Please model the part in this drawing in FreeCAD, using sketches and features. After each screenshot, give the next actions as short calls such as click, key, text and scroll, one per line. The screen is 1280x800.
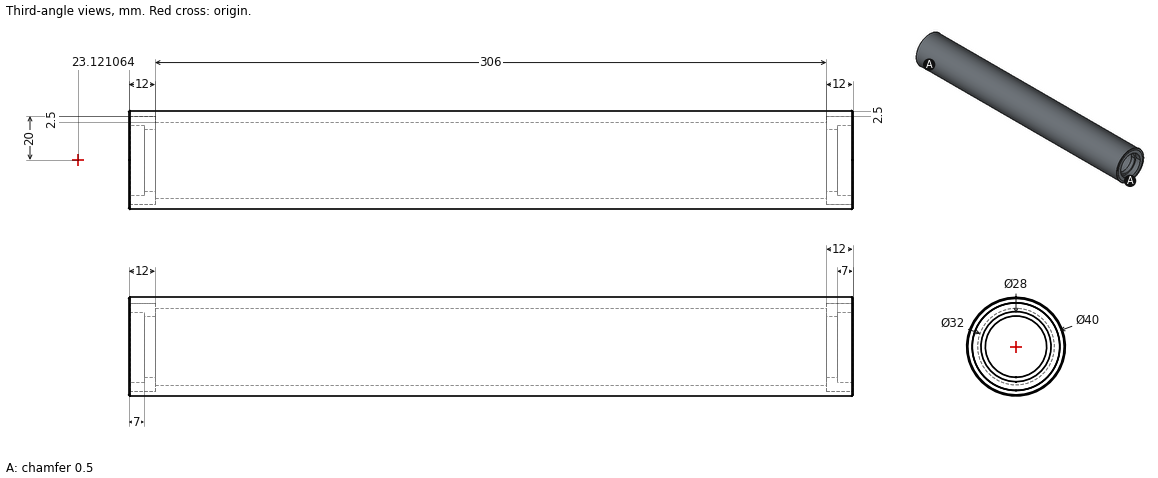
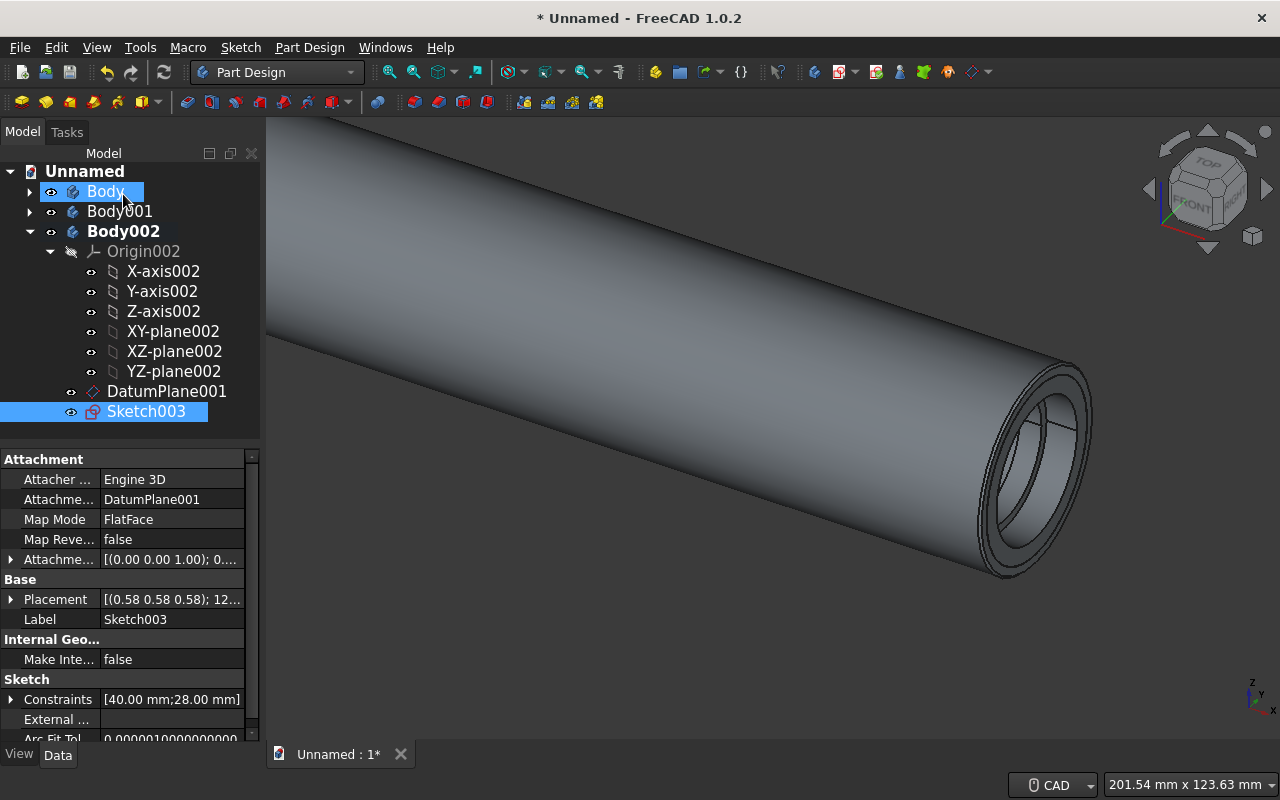
click(22, 102)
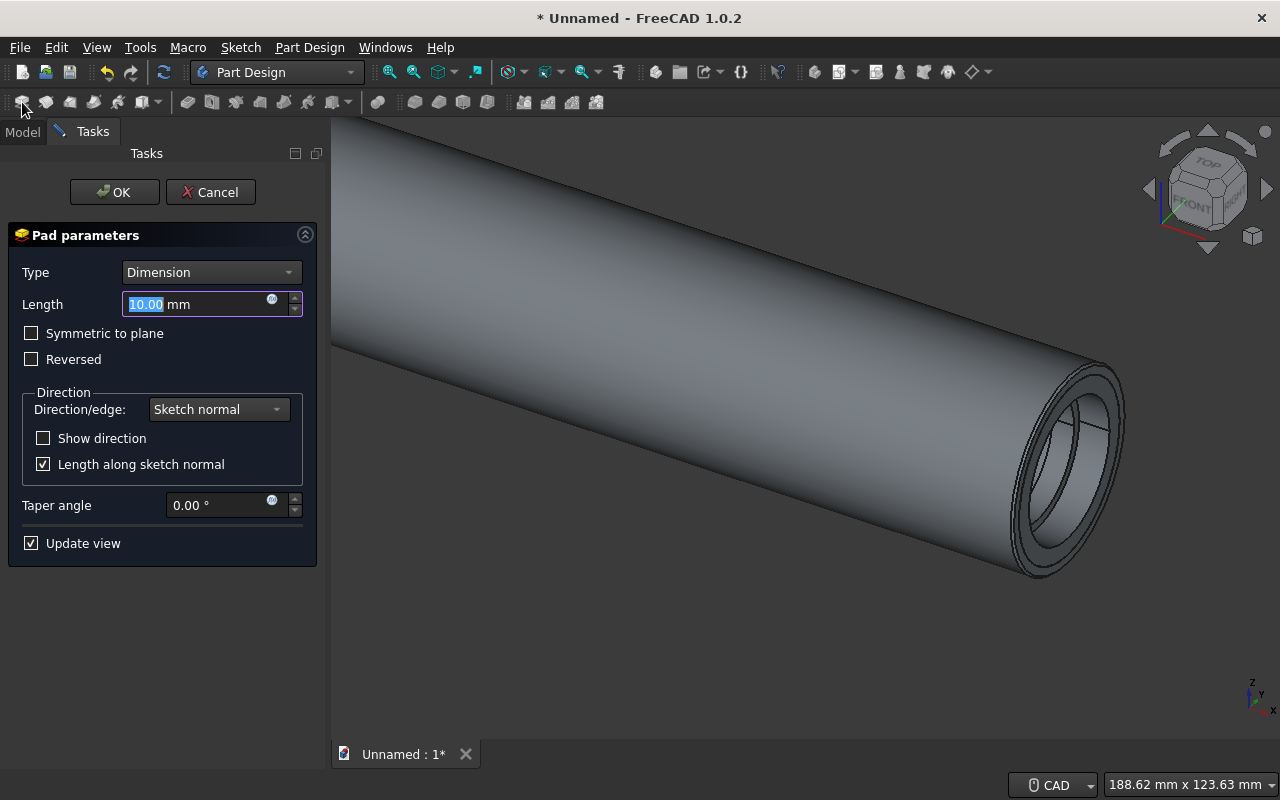
text(12)
key(Tab)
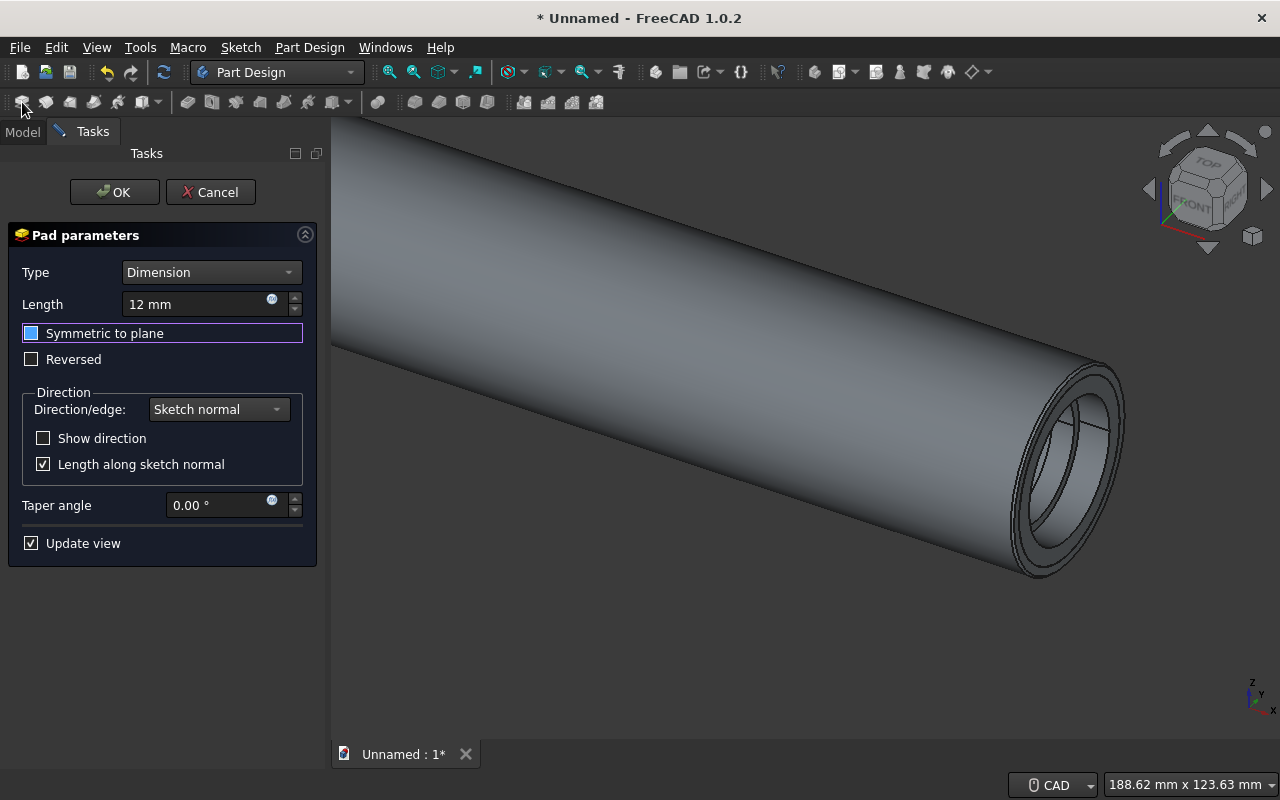
click(30, 359)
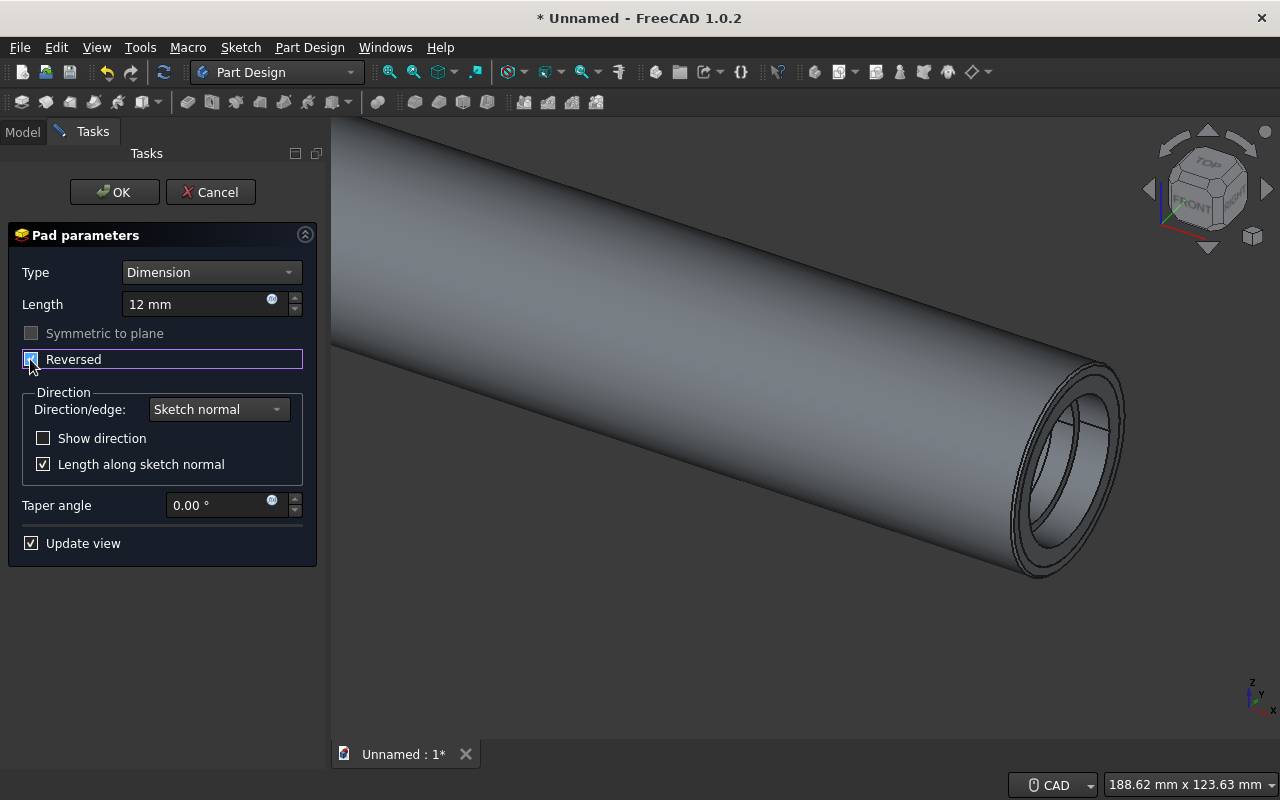
click(115, 192)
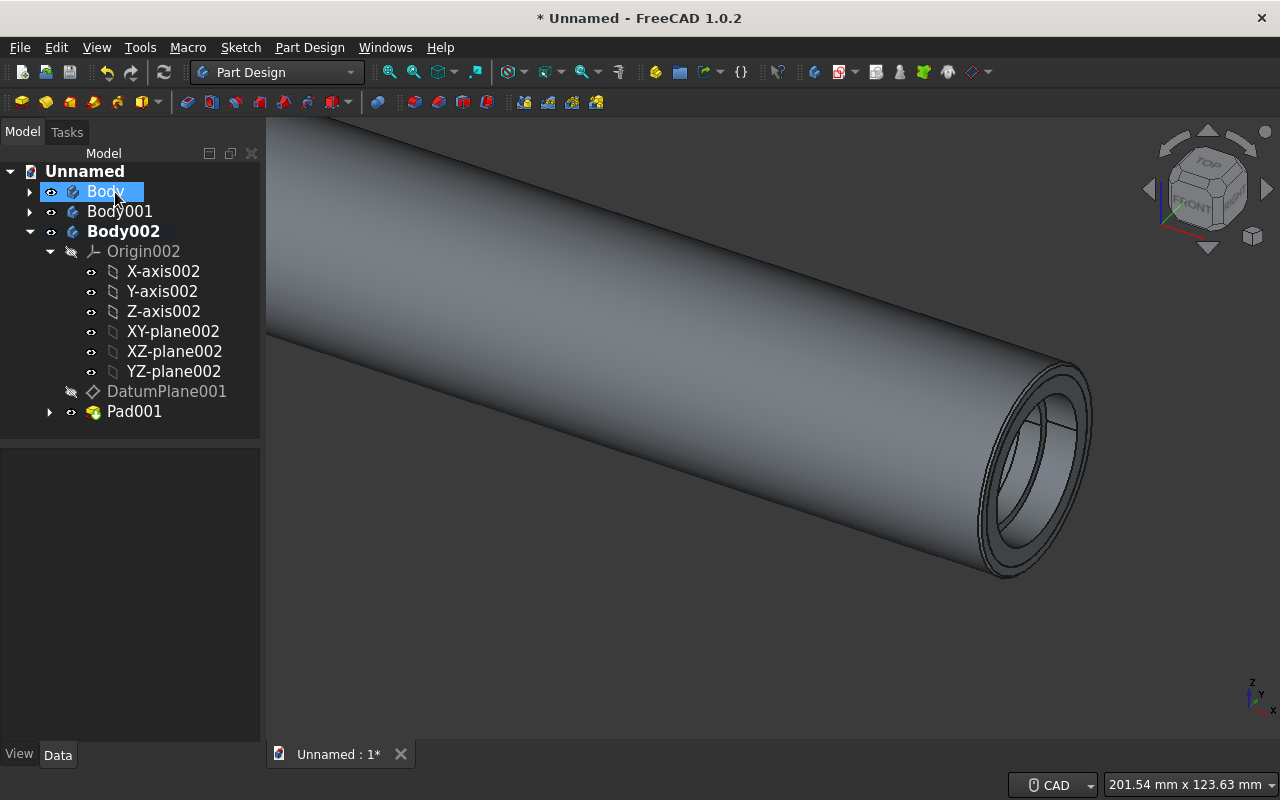
click(390, 72)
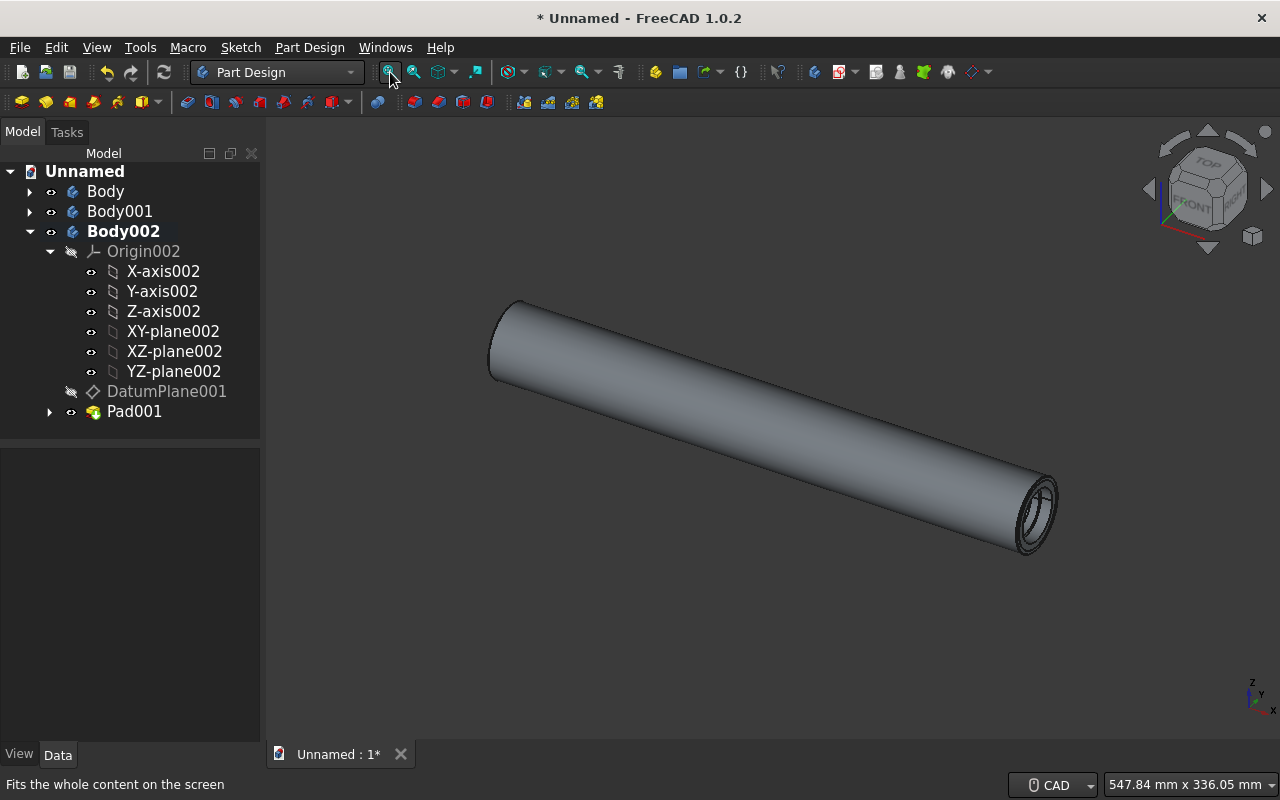
key(6)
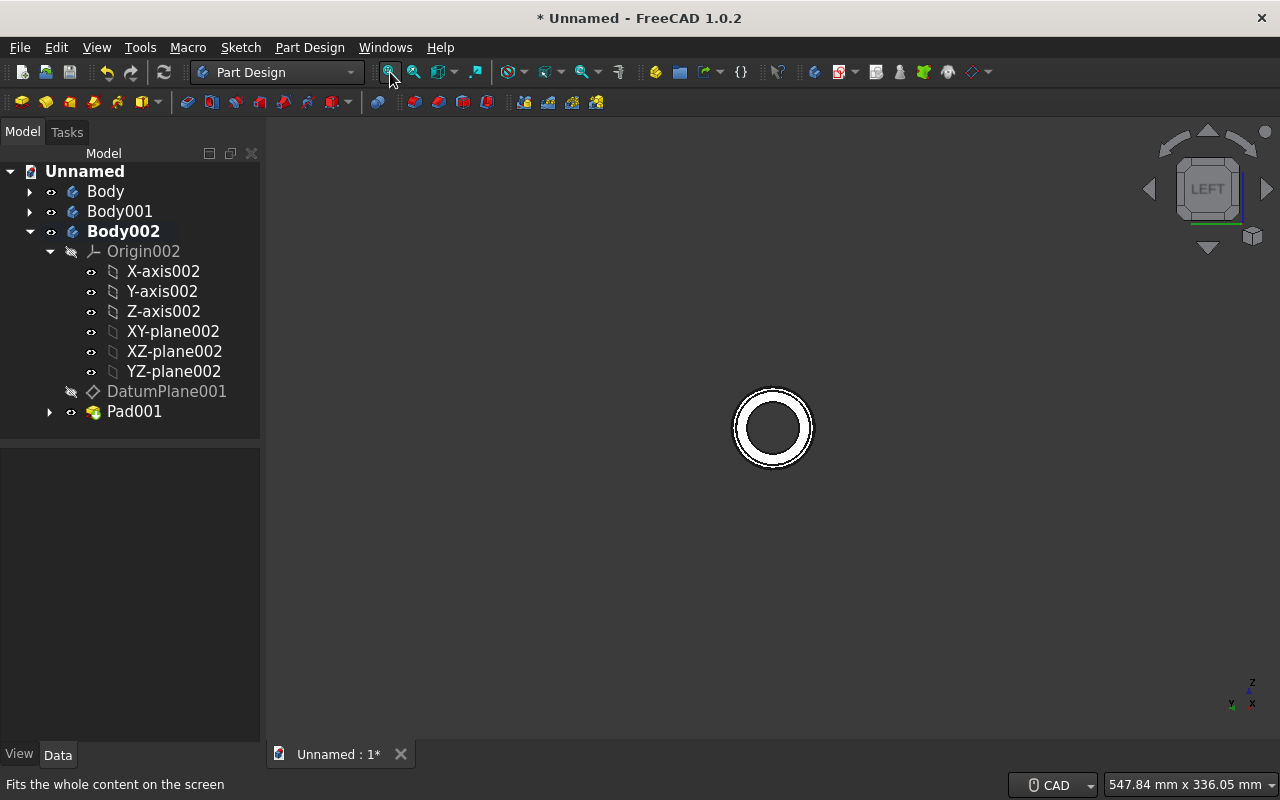
click(390, 72)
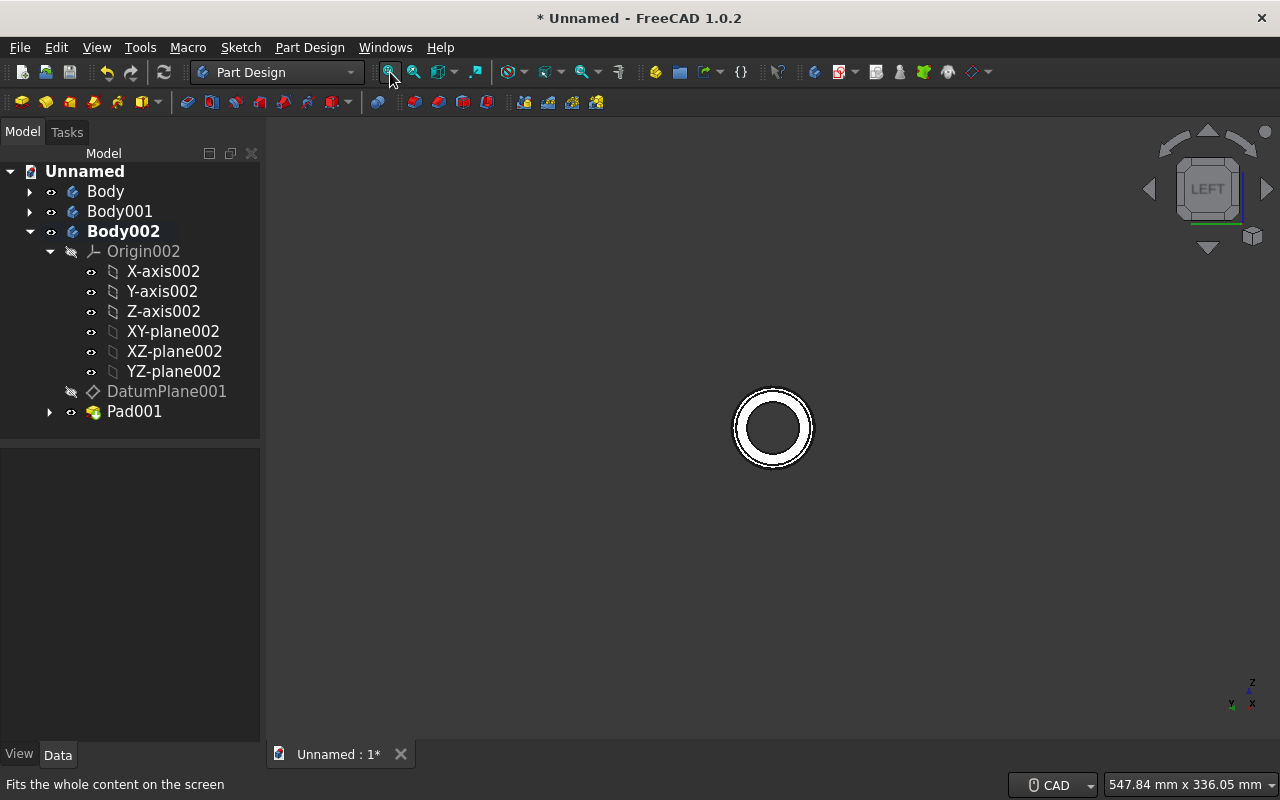
scroll(773, 459, up, 5)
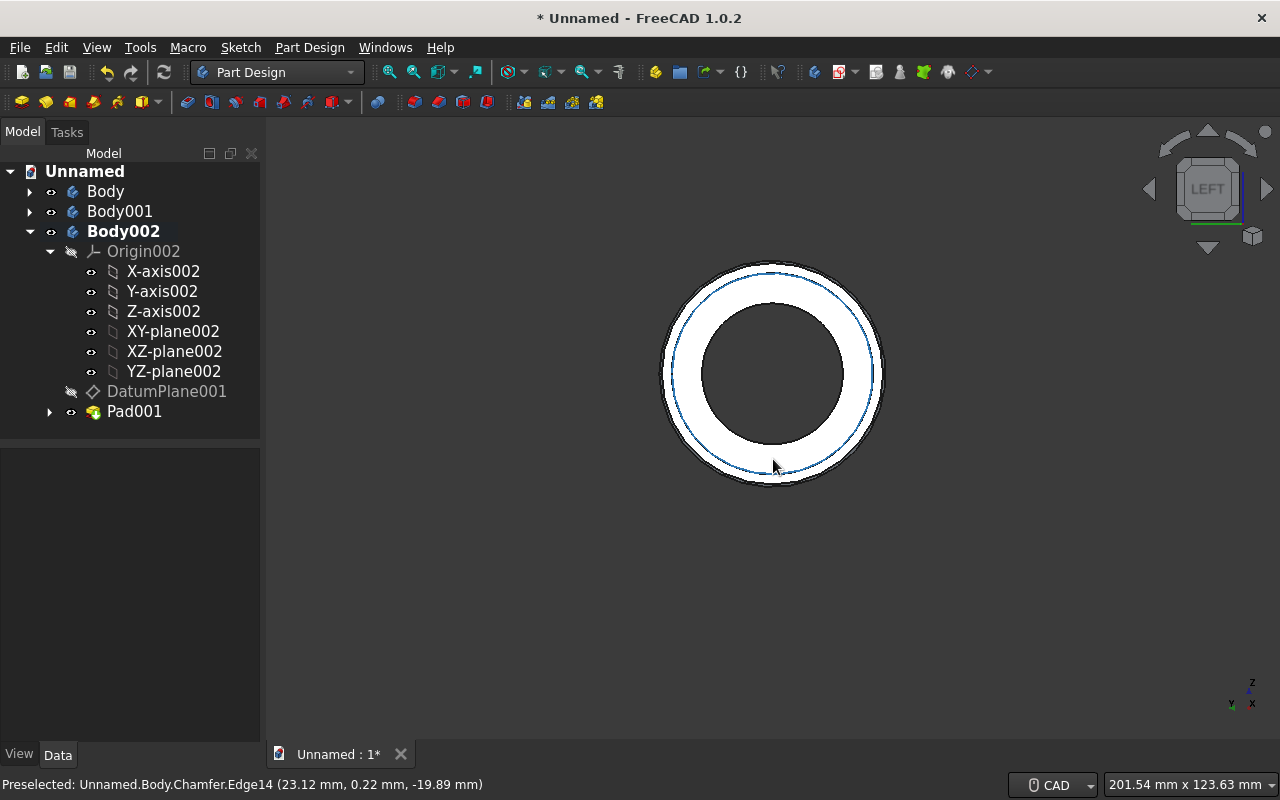
click(772, 459)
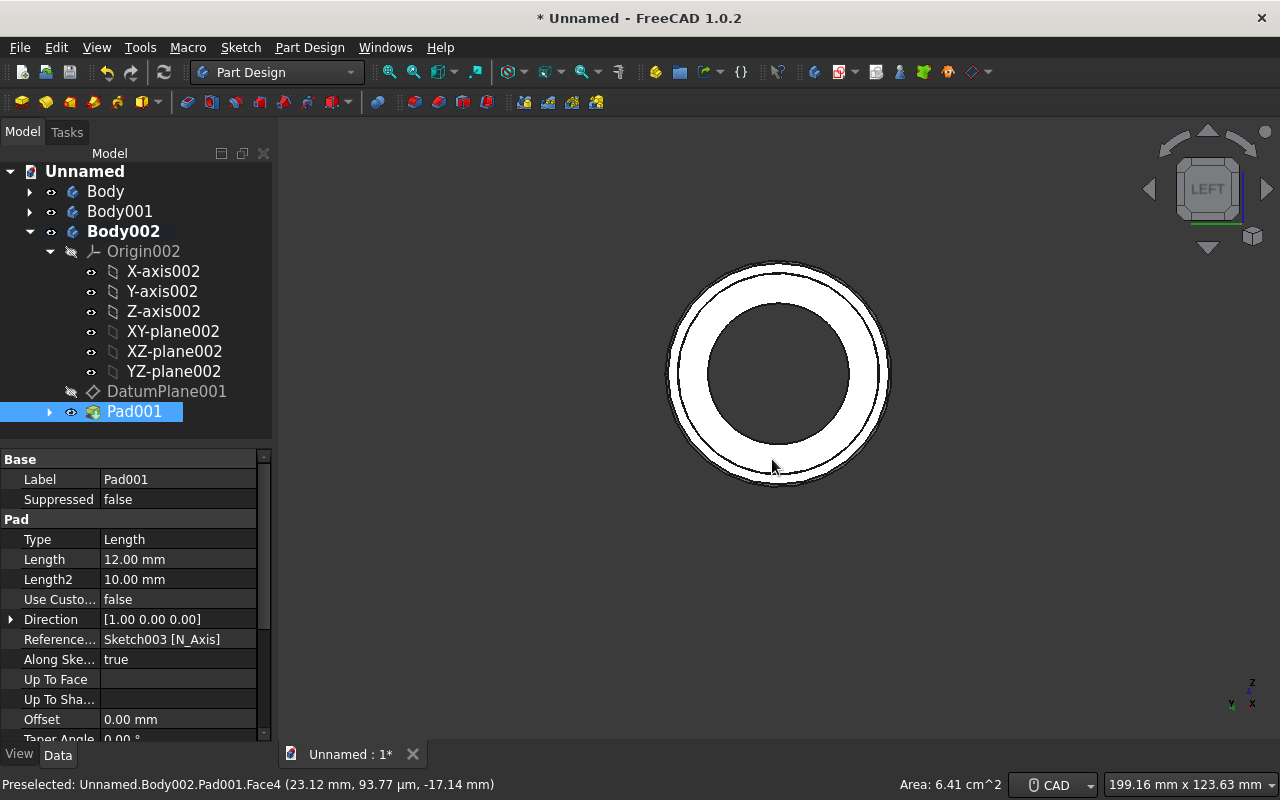
click(840, 72)